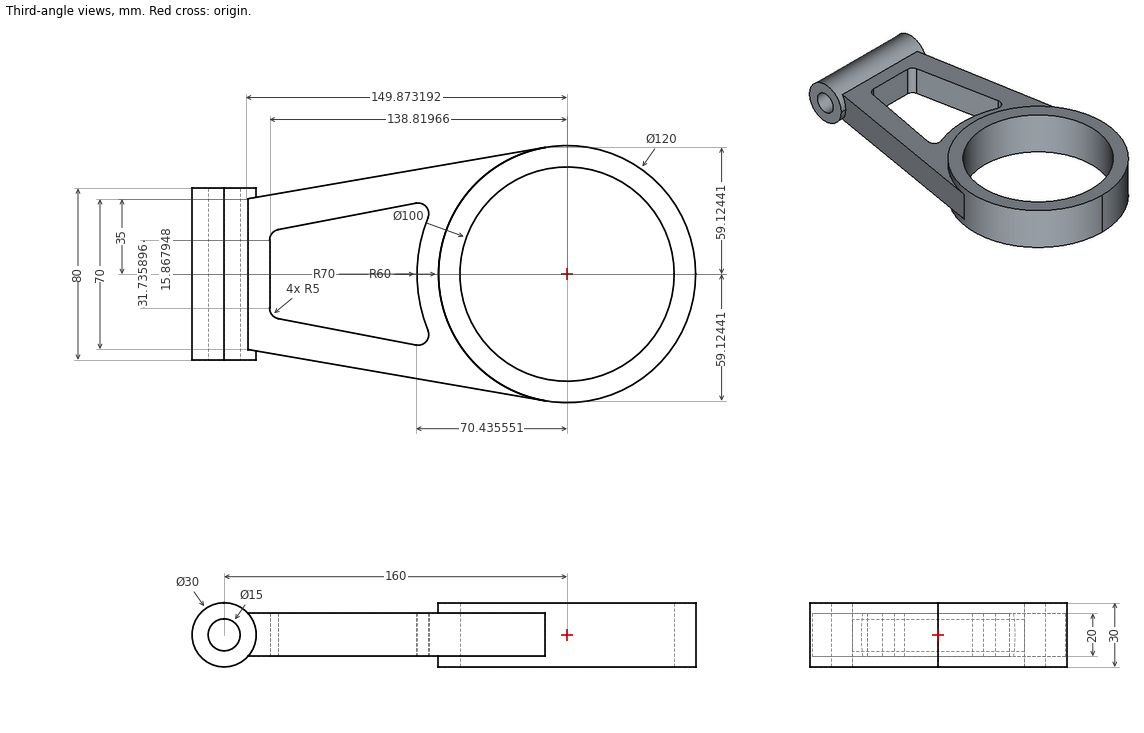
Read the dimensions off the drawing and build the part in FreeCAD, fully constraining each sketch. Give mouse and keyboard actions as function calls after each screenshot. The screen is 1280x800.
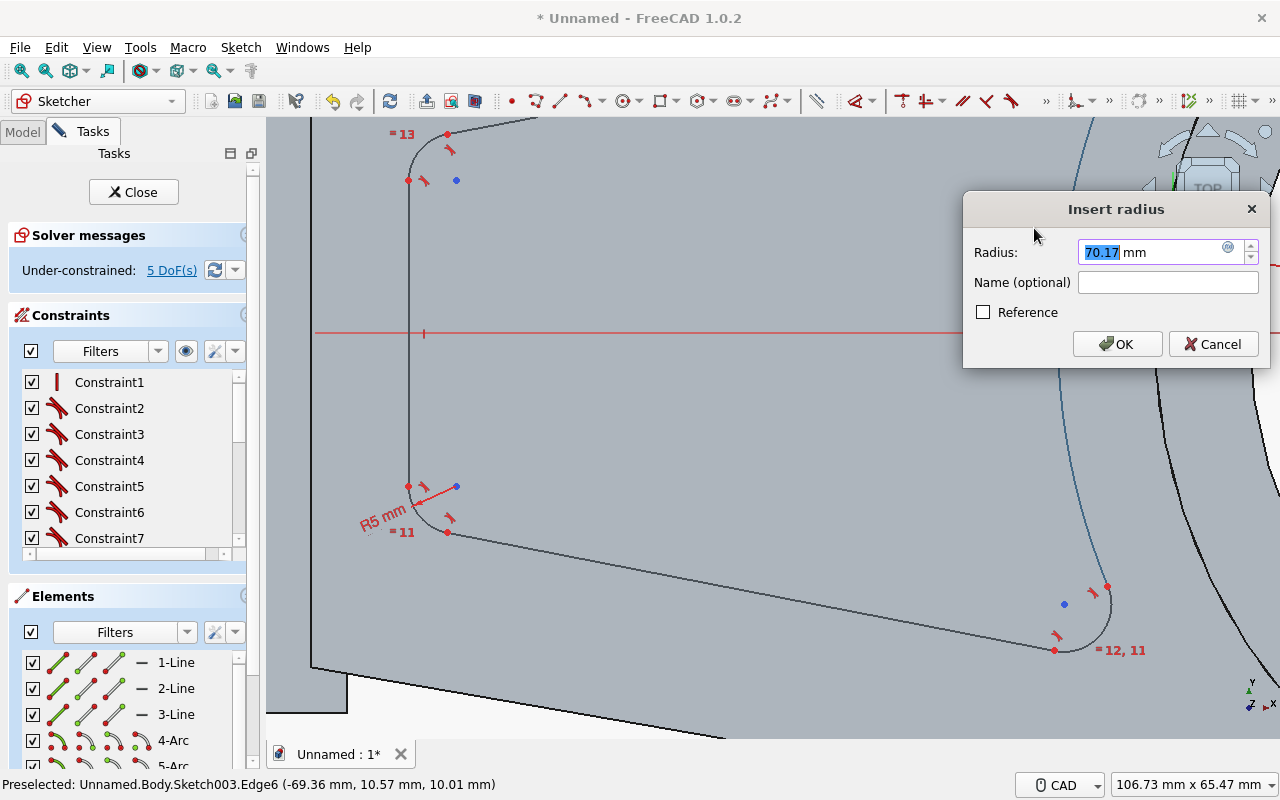
text(70)
key(Return)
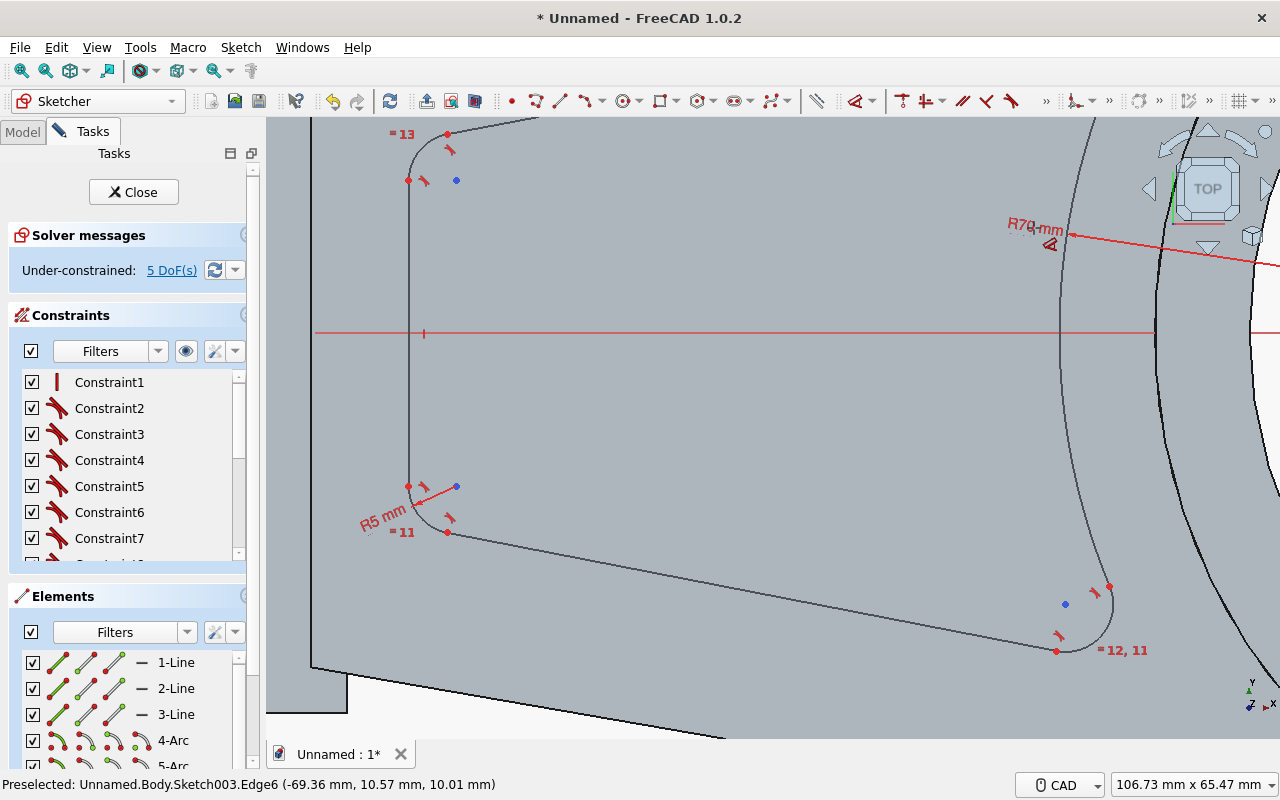
click(409, 272)
click(375, 263)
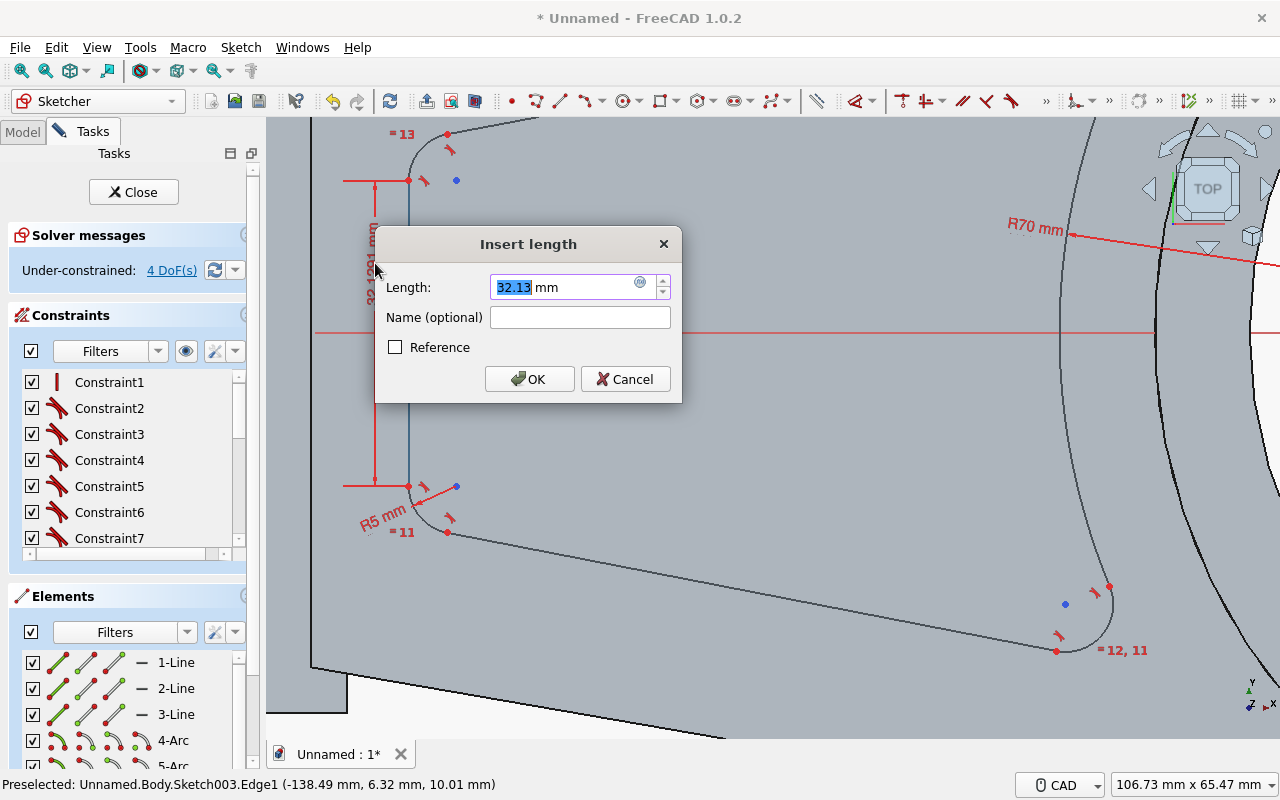
text(31.735896)
key(Return)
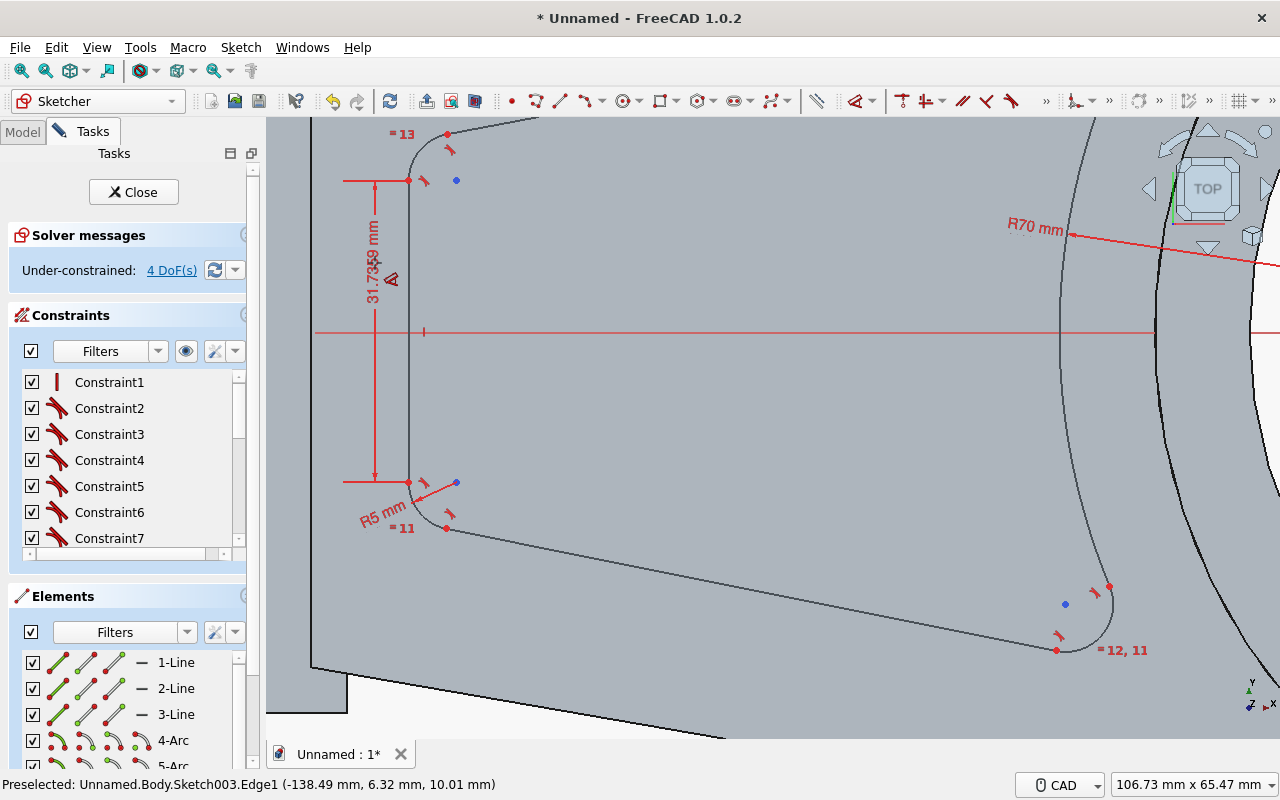
click(409, 181)
click(762, 147)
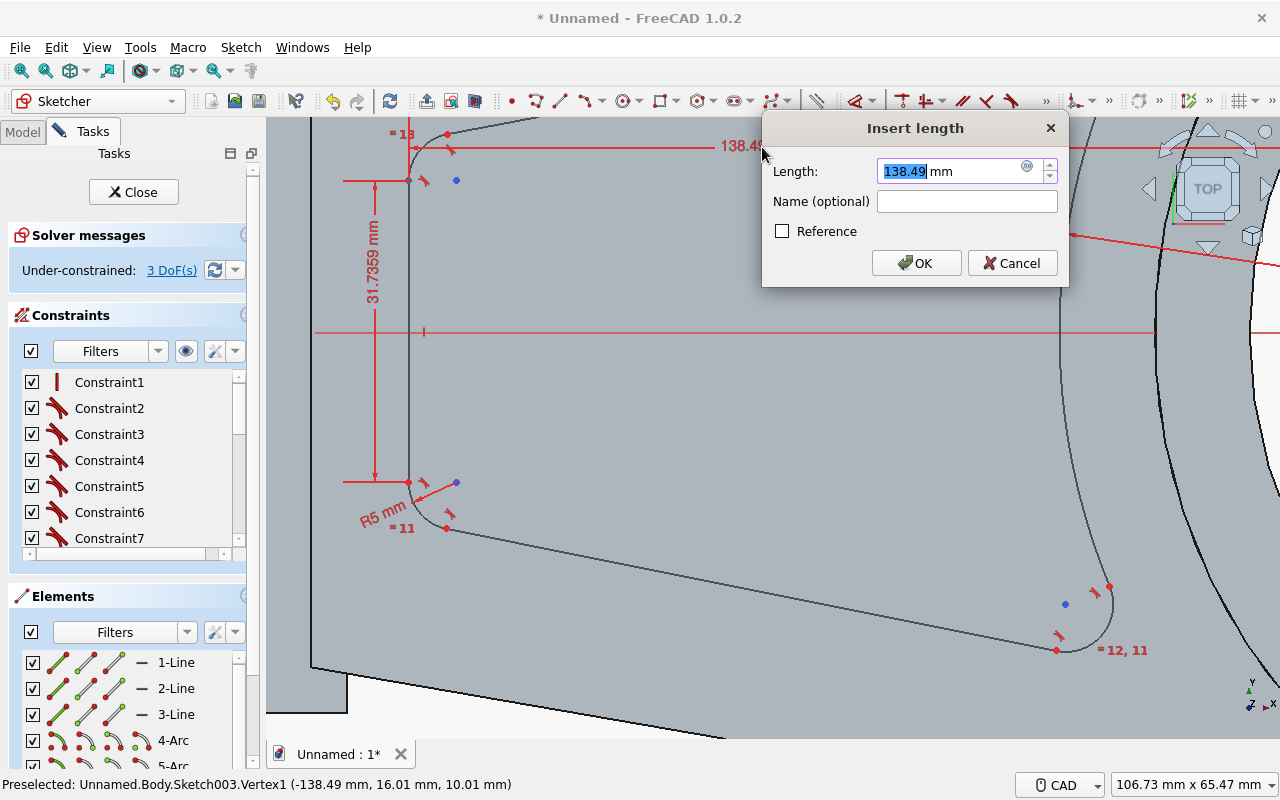
text(138.81966)
key(Return)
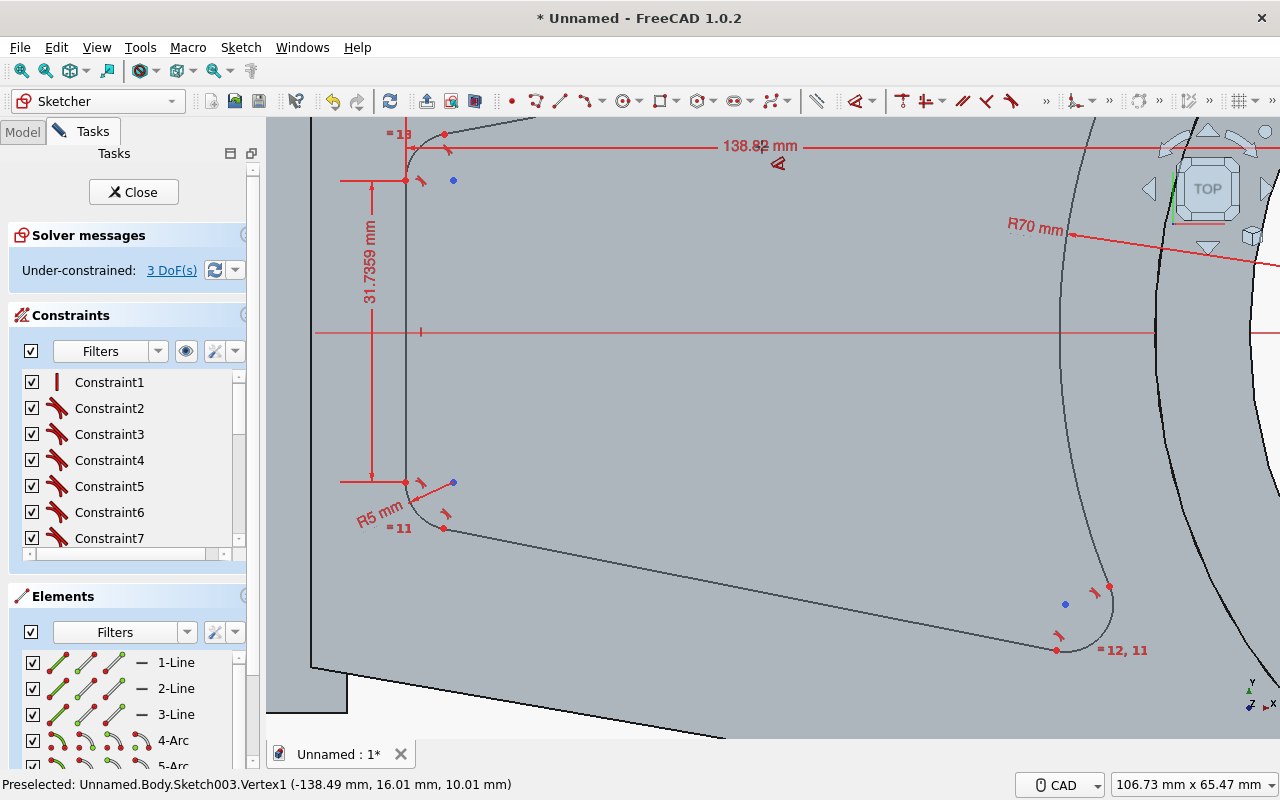
click(406, 181)
click(372, 222)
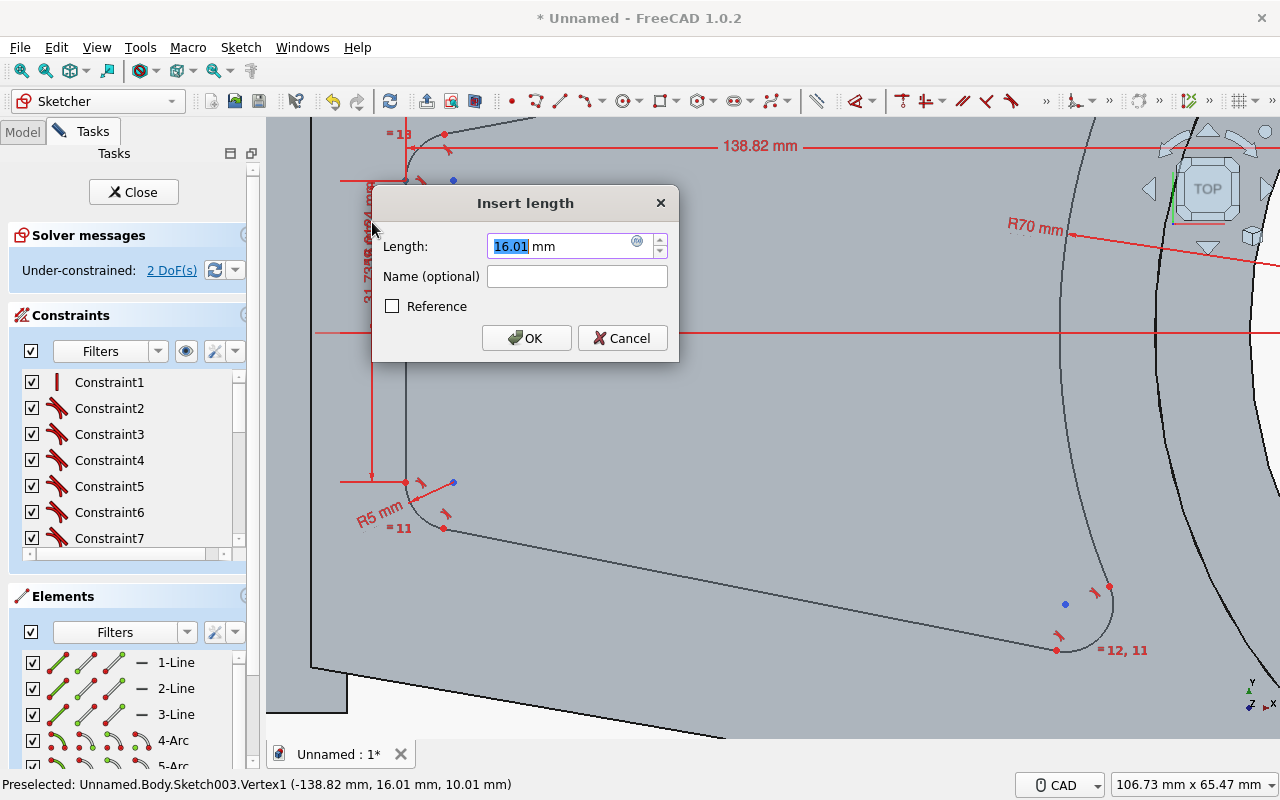
text(15.867948)
key(Return)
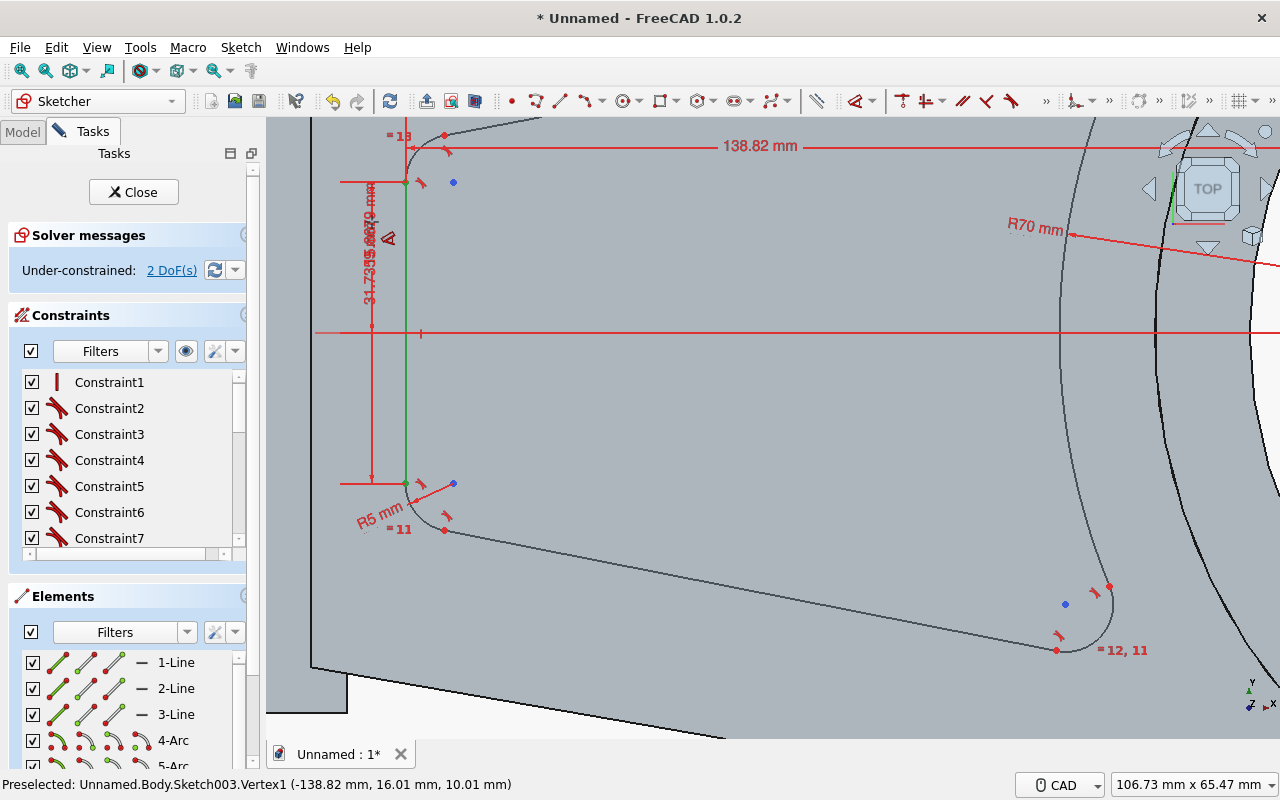
click(1057, 651)
click(1086, 685)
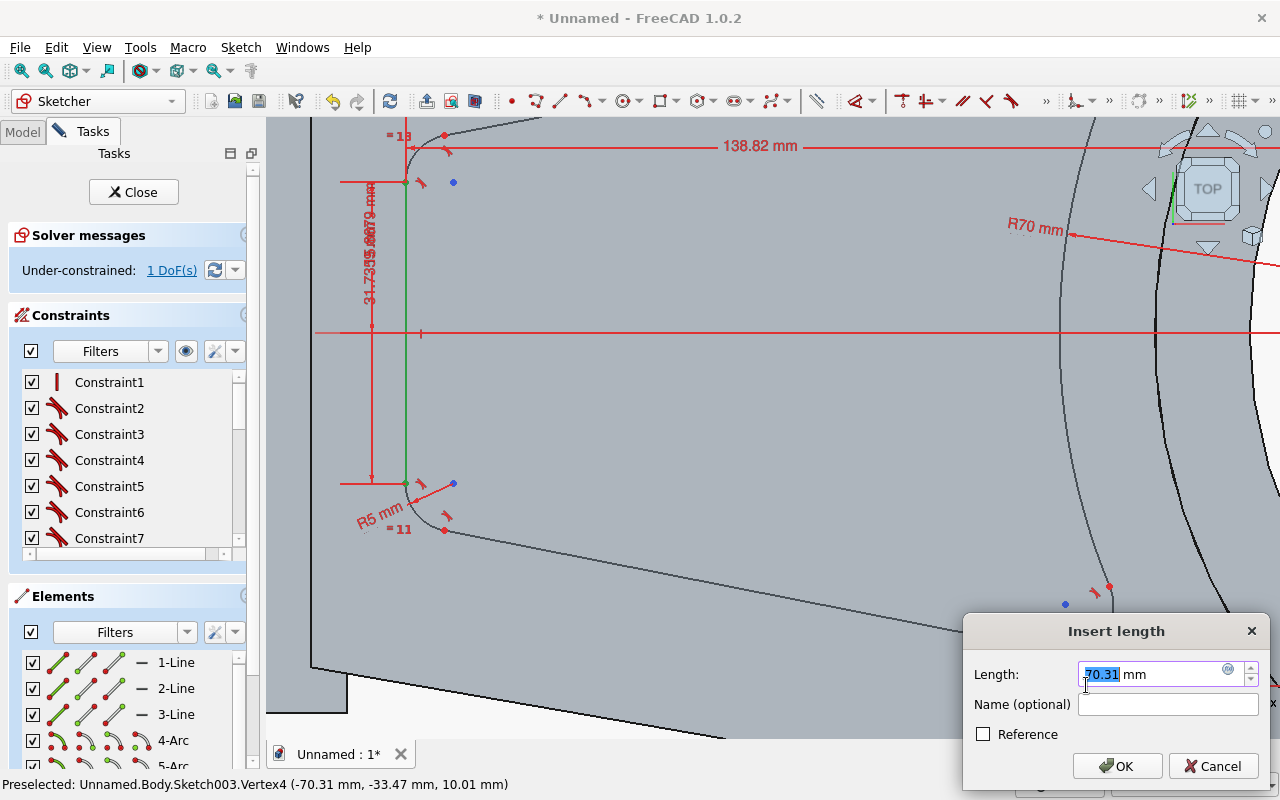
text(70.435551)
key(Return)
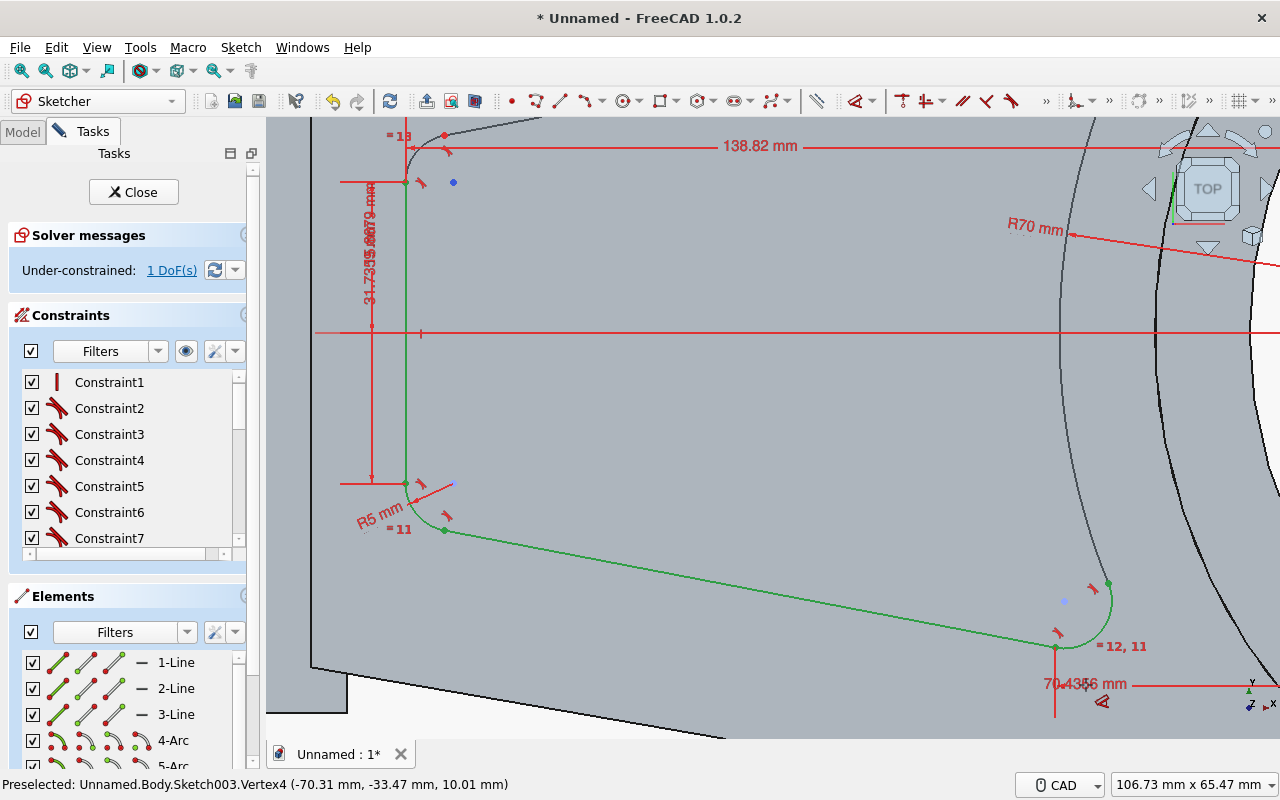
scroll(410, 506, down, 4)